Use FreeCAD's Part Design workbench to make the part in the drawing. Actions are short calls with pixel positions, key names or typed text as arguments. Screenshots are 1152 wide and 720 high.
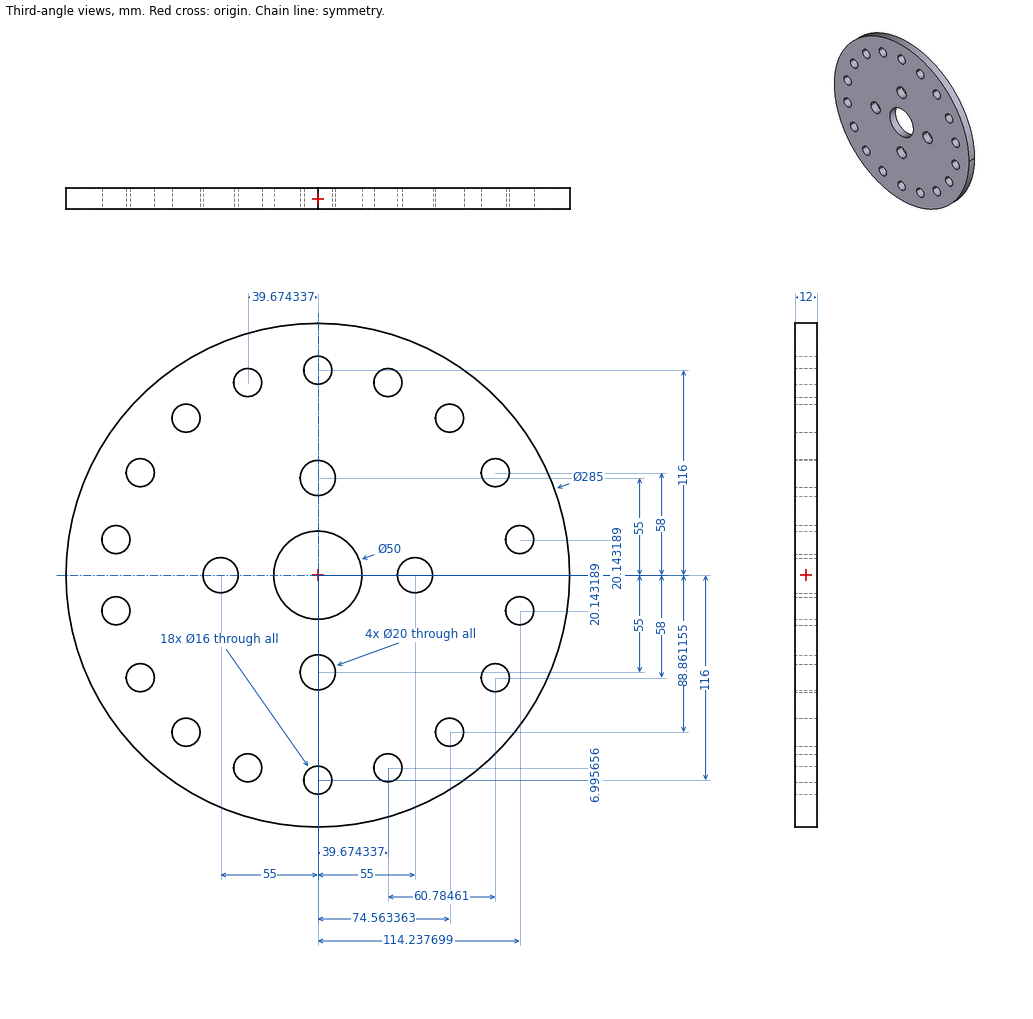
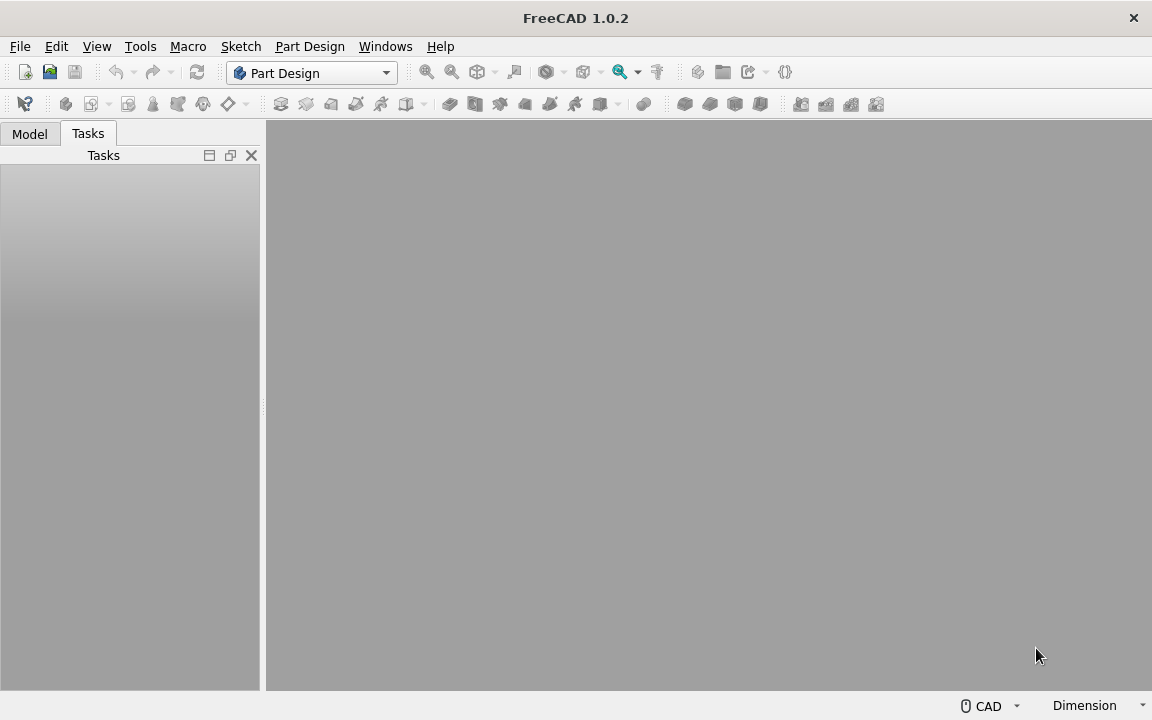
click(25, 72)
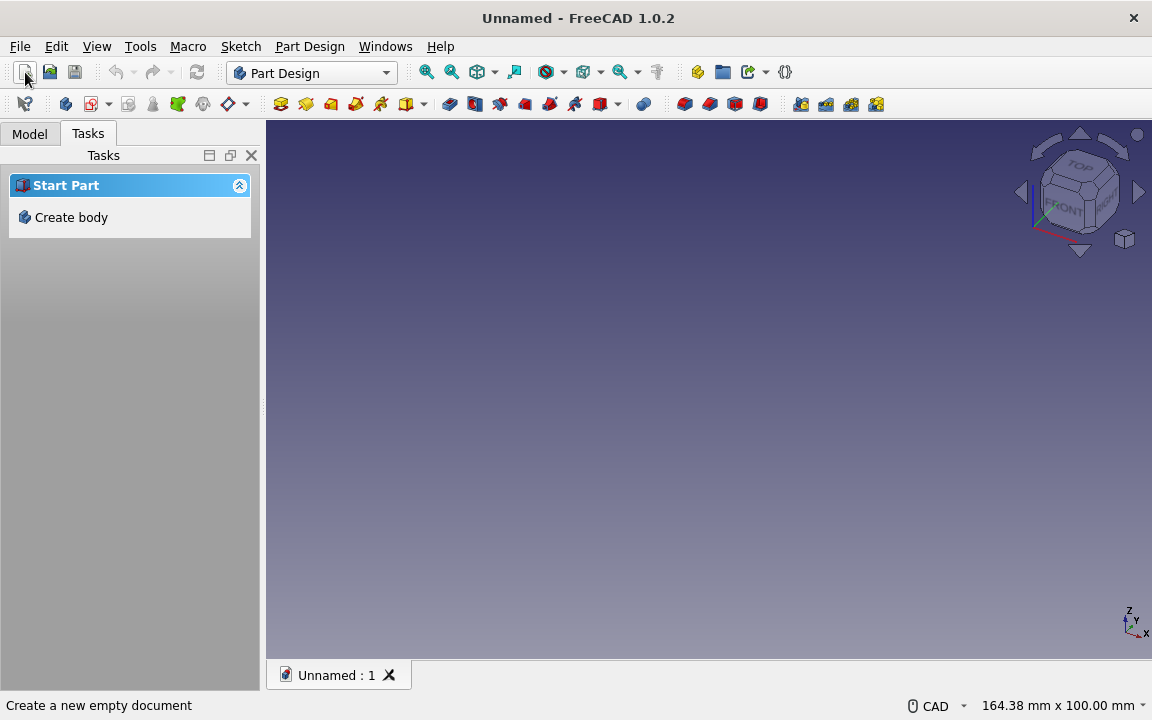
click(90, 104)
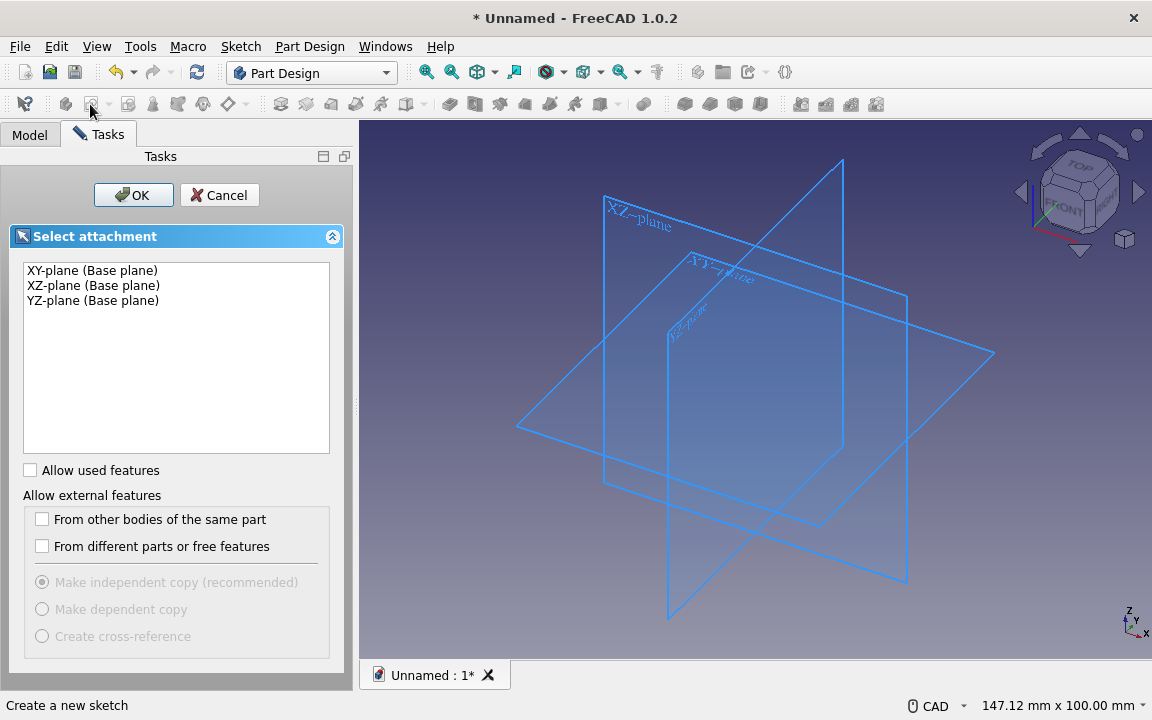
click(84, 286)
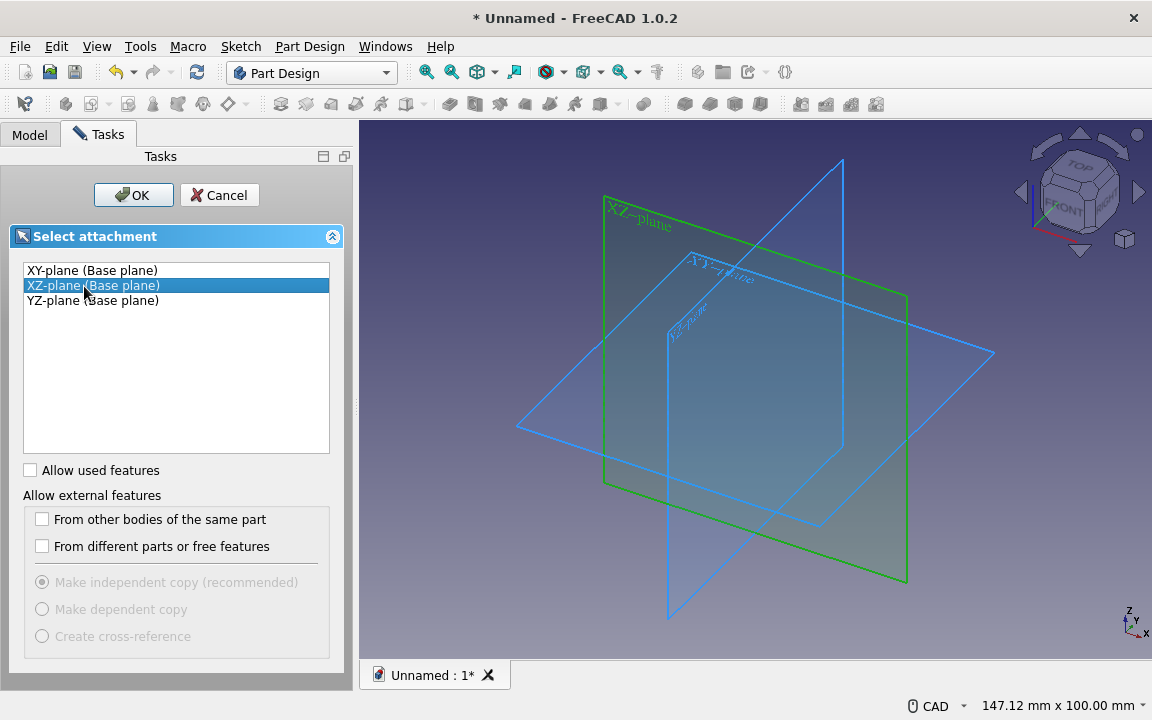
click(134, 195)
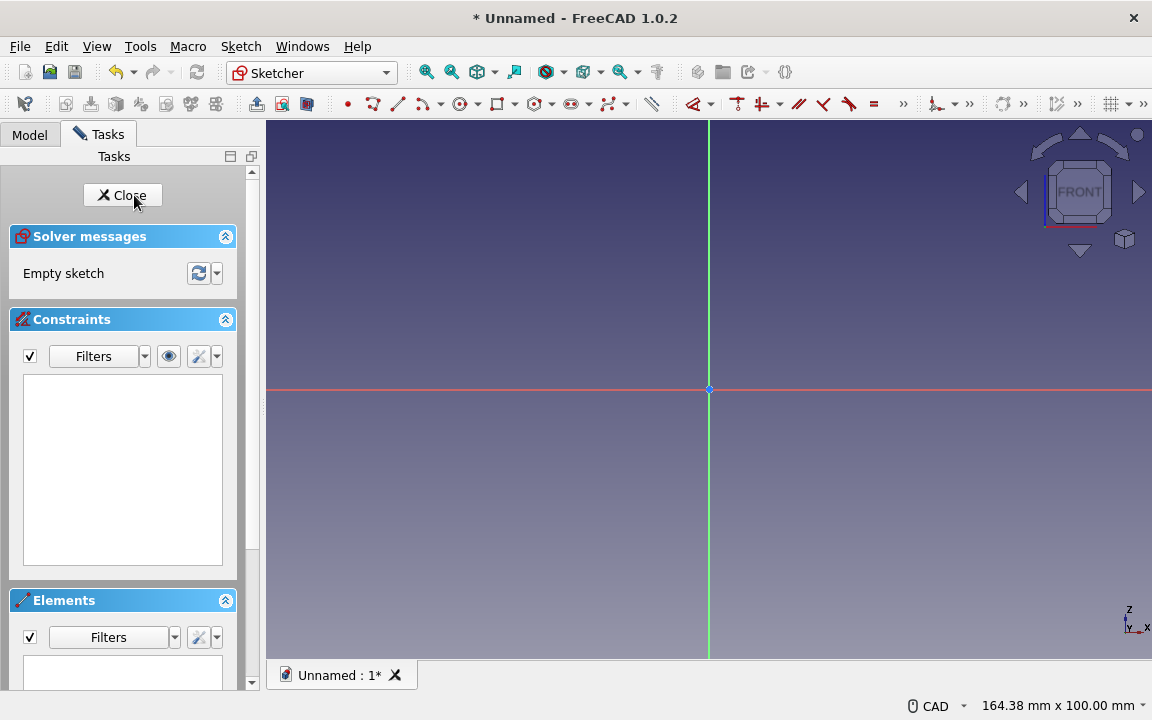
scroll(623, 389, down, 8)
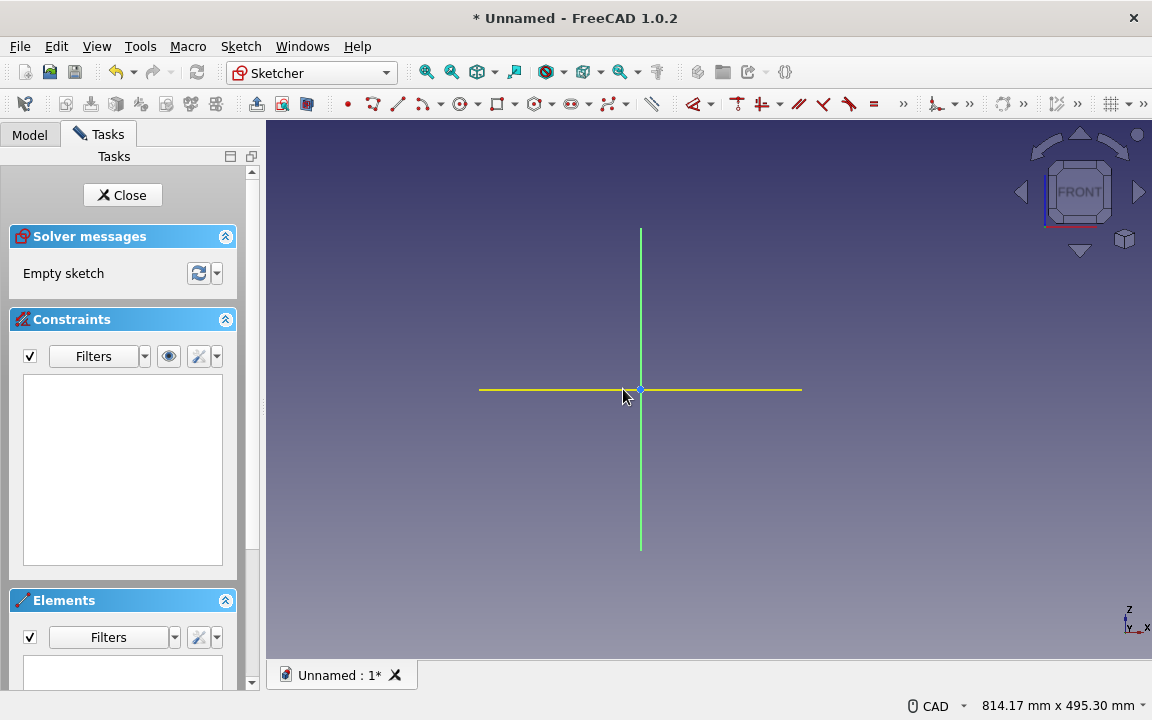
click(460, 104)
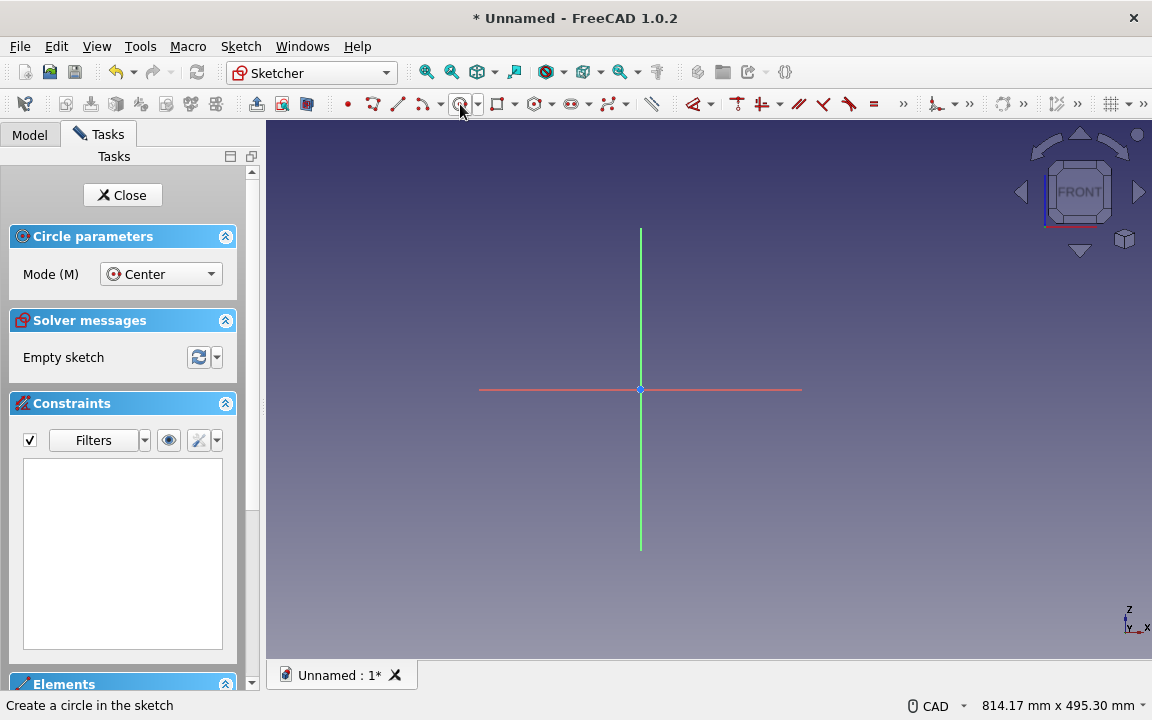
click(641, 390)
move(750, 280)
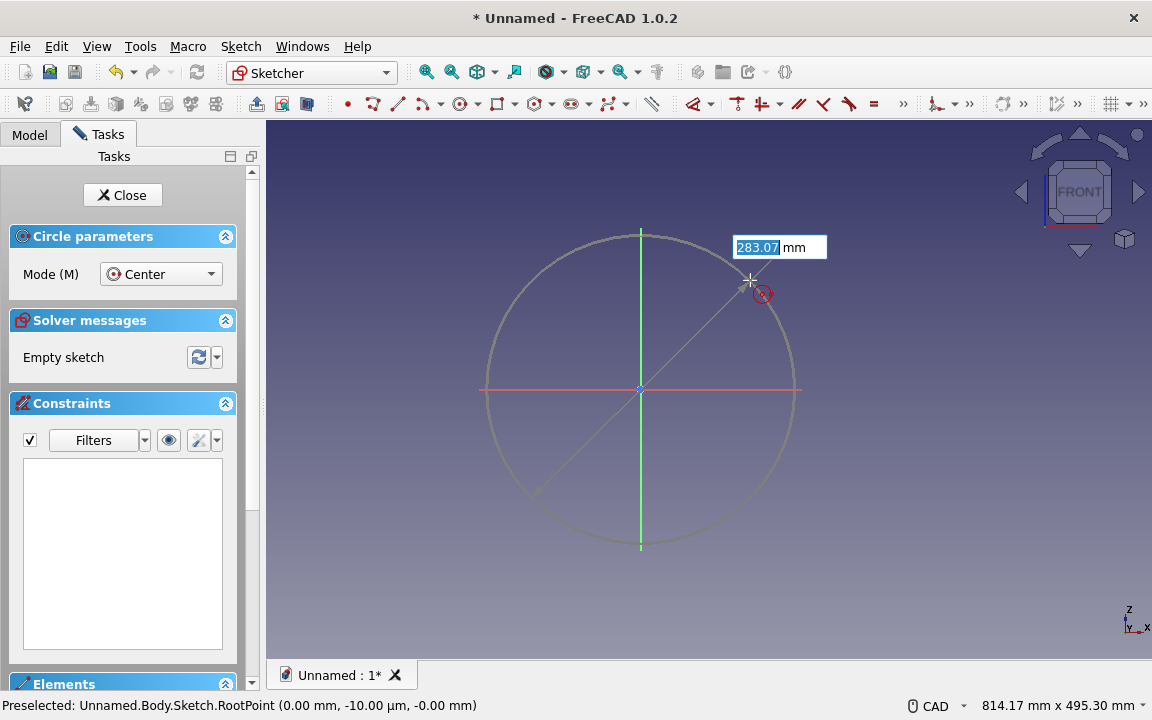
text(285)
key(Return)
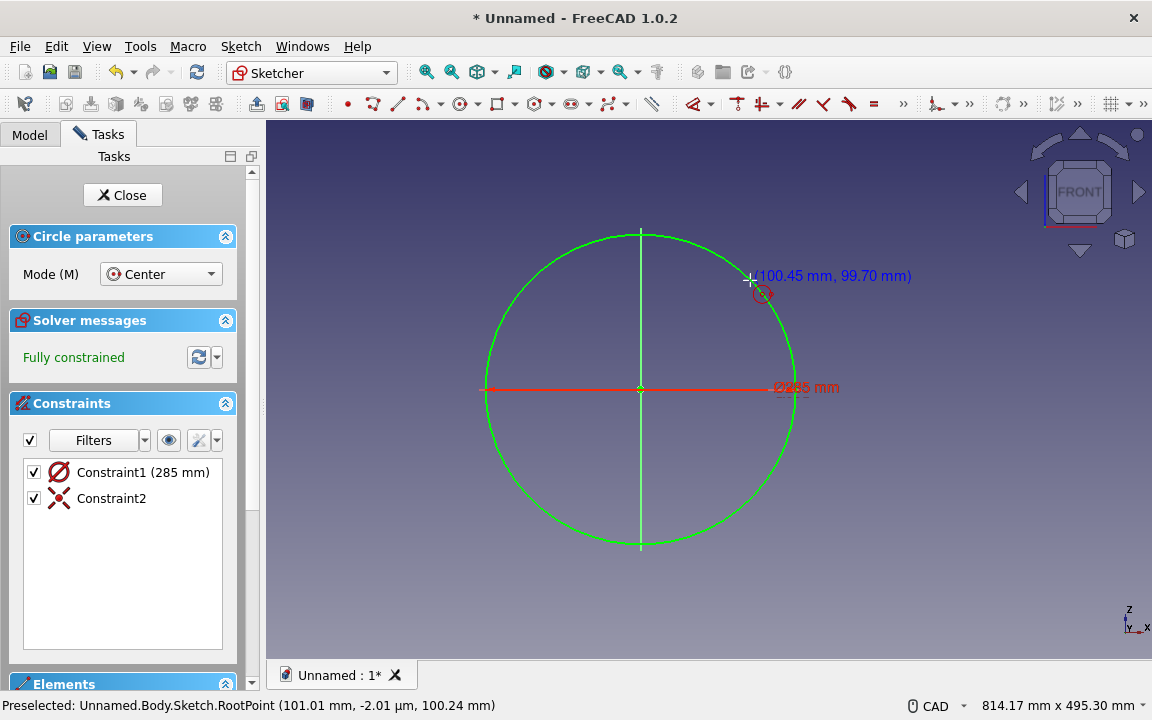
click(641, 390)
move(660, 370)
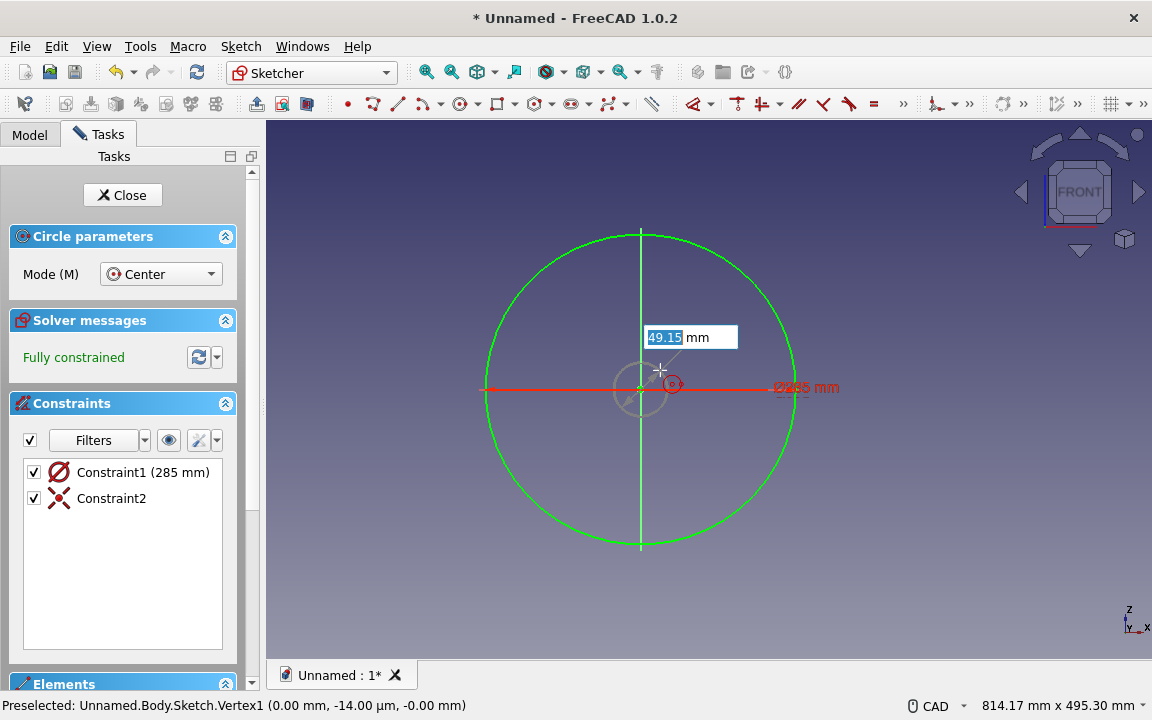
text(50)
key(Return)
key(Escape)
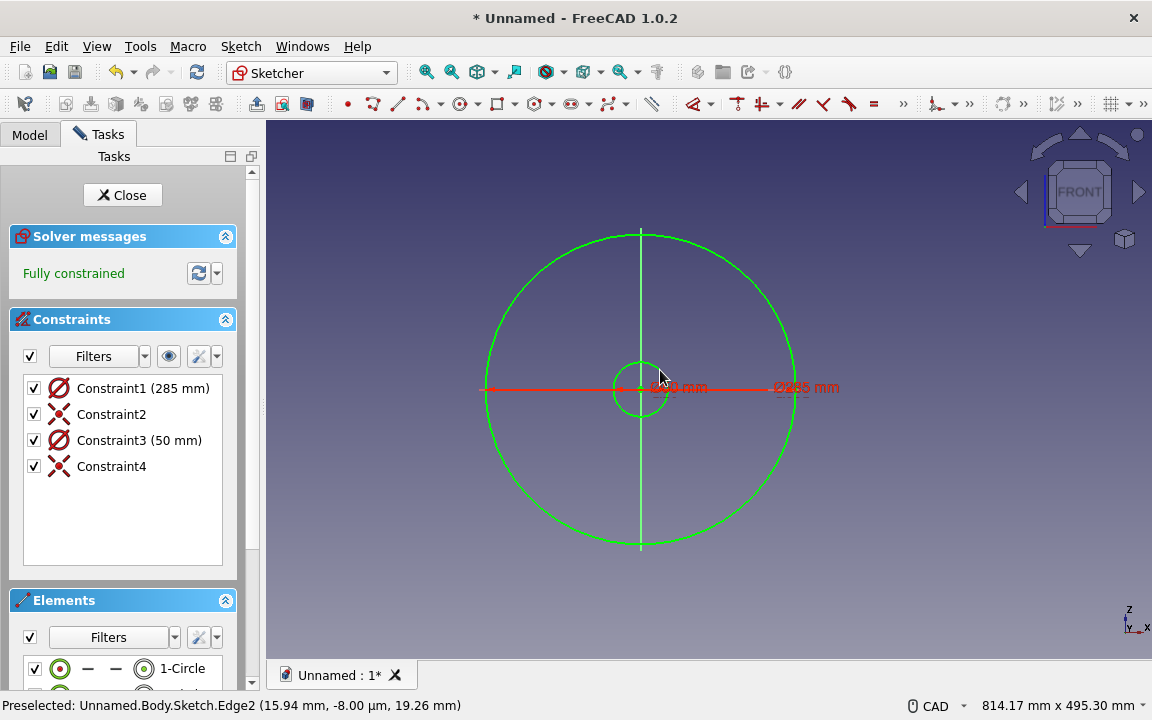
click(123, 195)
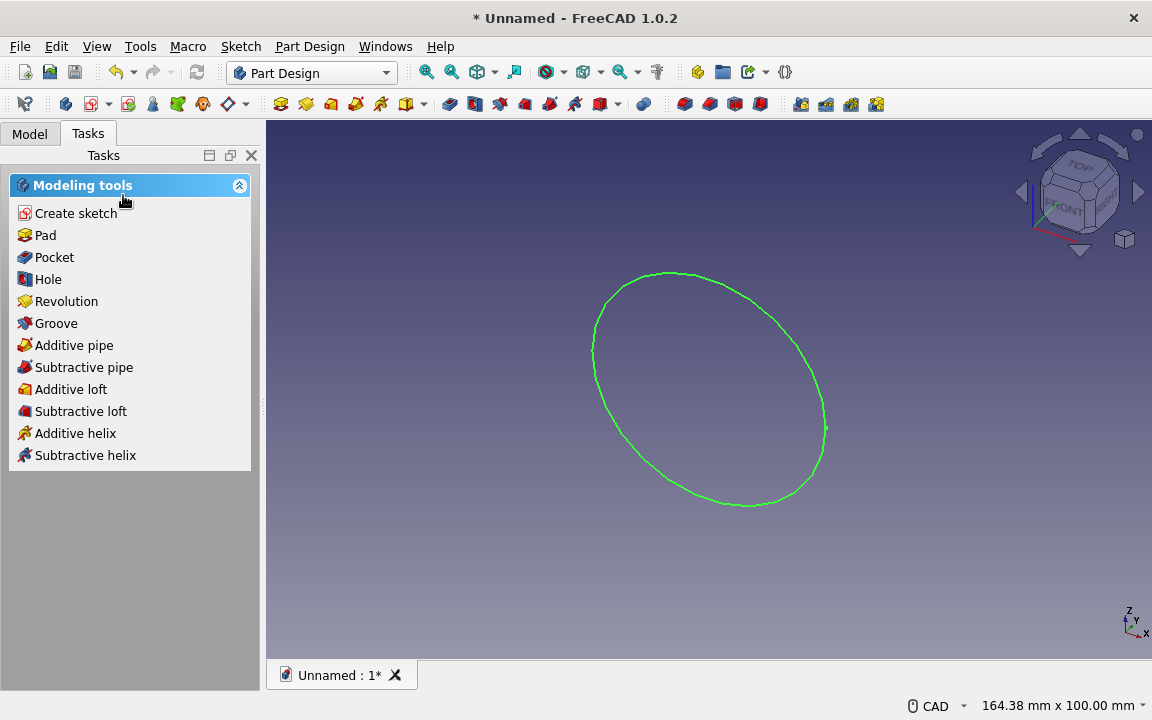
click(281, 104)